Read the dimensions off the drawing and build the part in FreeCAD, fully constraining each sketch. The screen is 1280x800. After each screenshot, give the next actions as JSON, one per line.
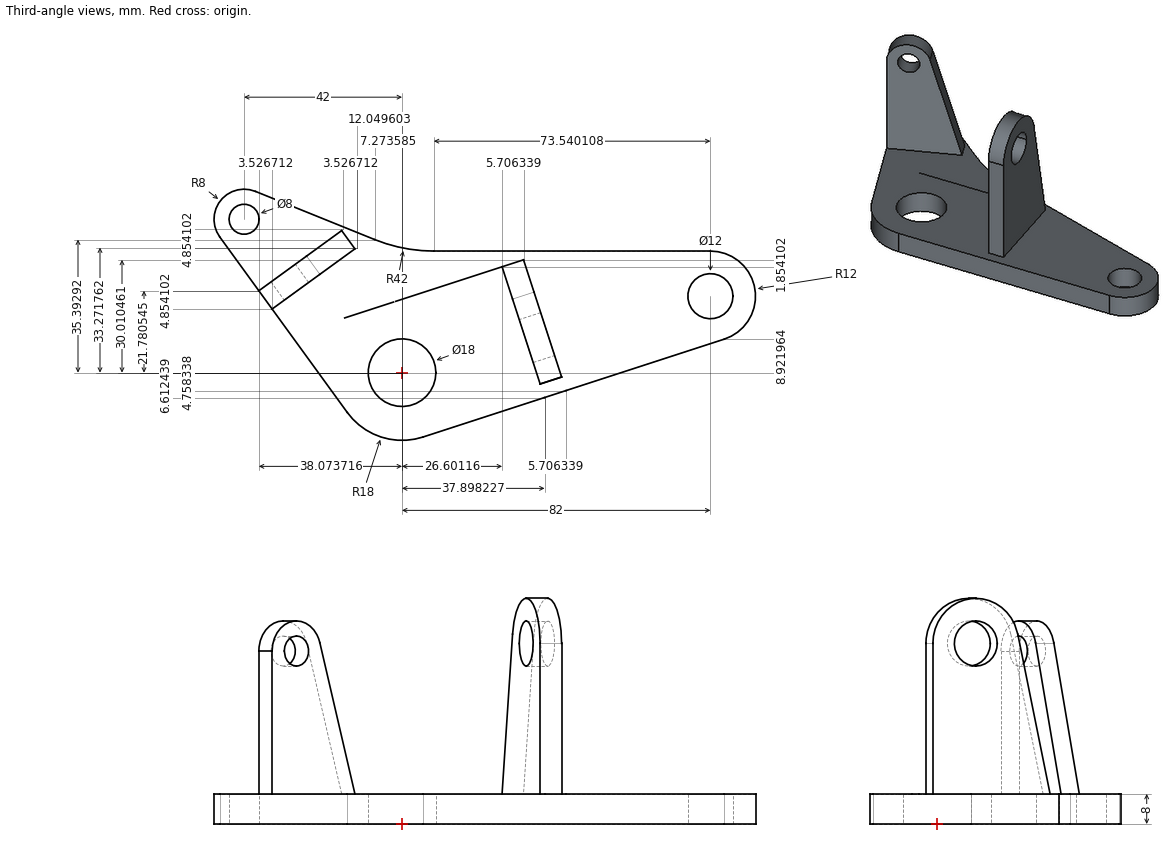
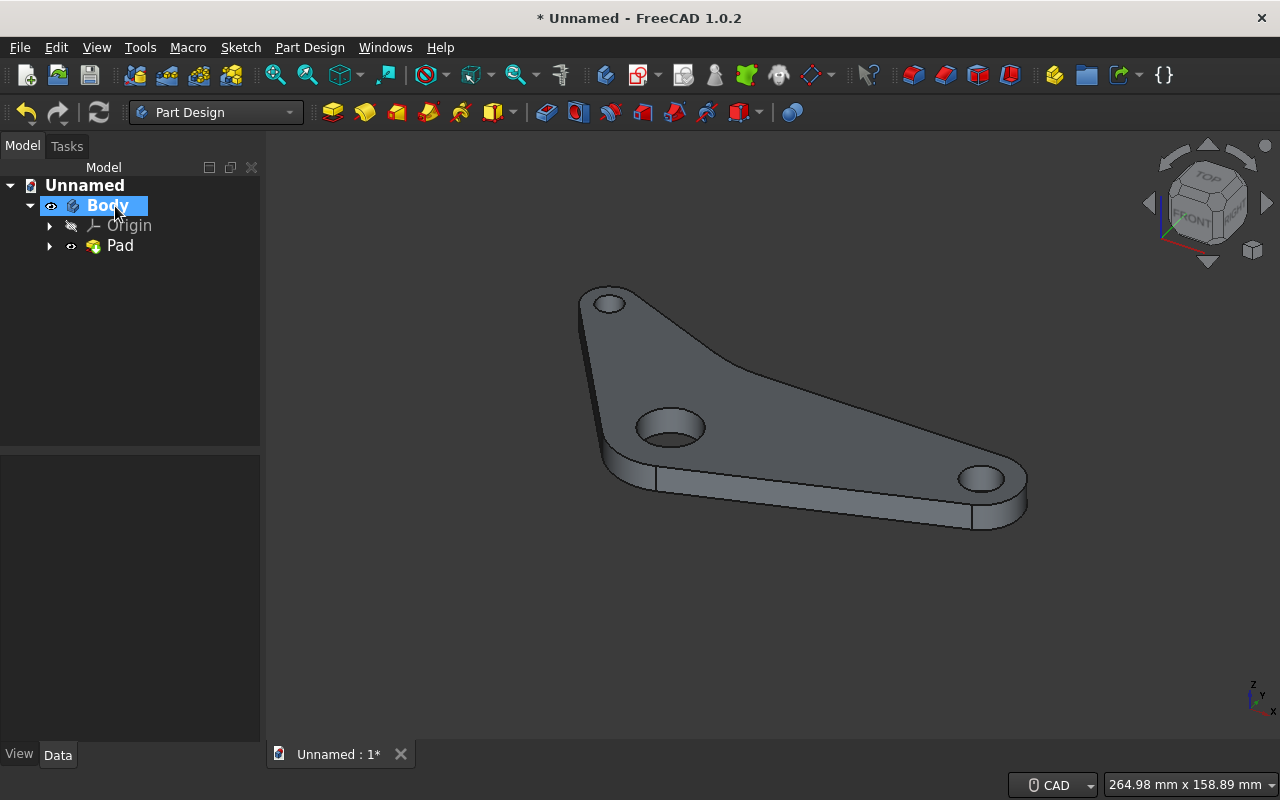
{"action": "left_click", "coordinate": [841, 444]}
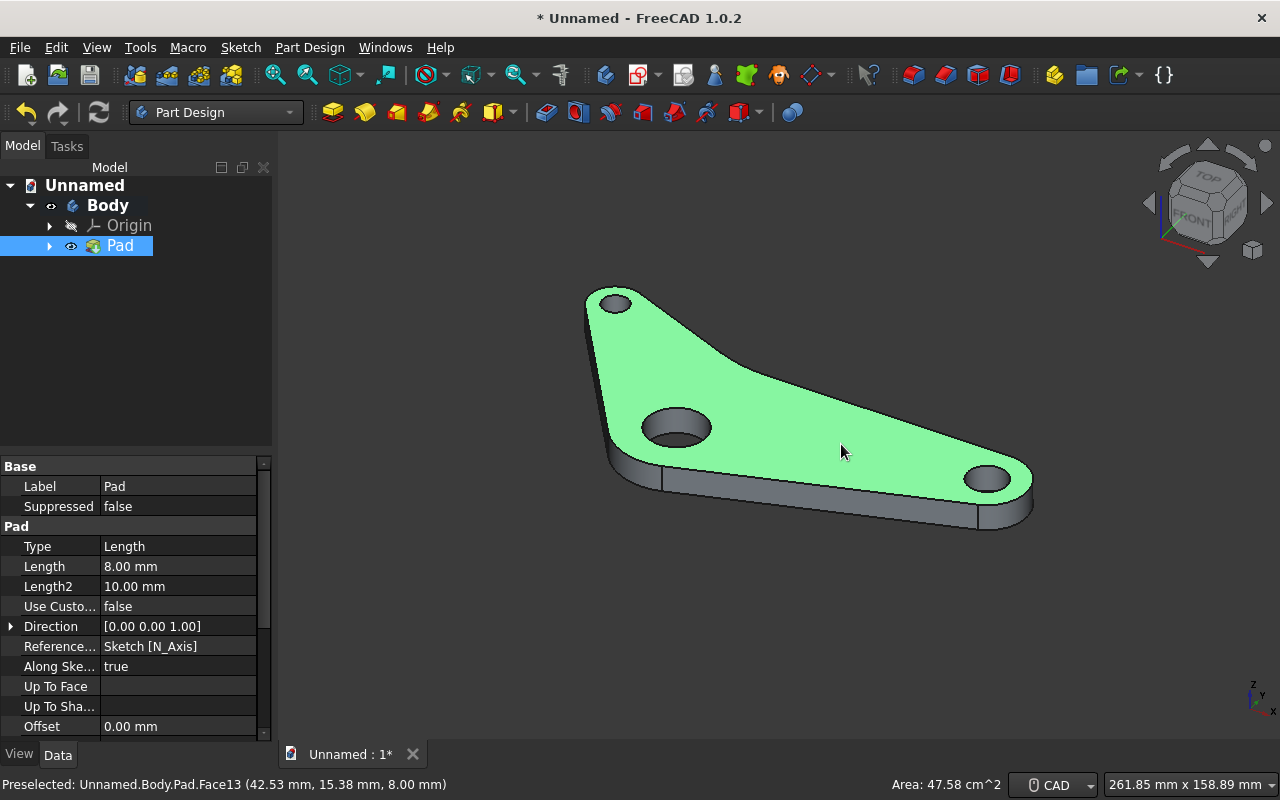
{"action": "left_click", "coordinate": [638, 76]}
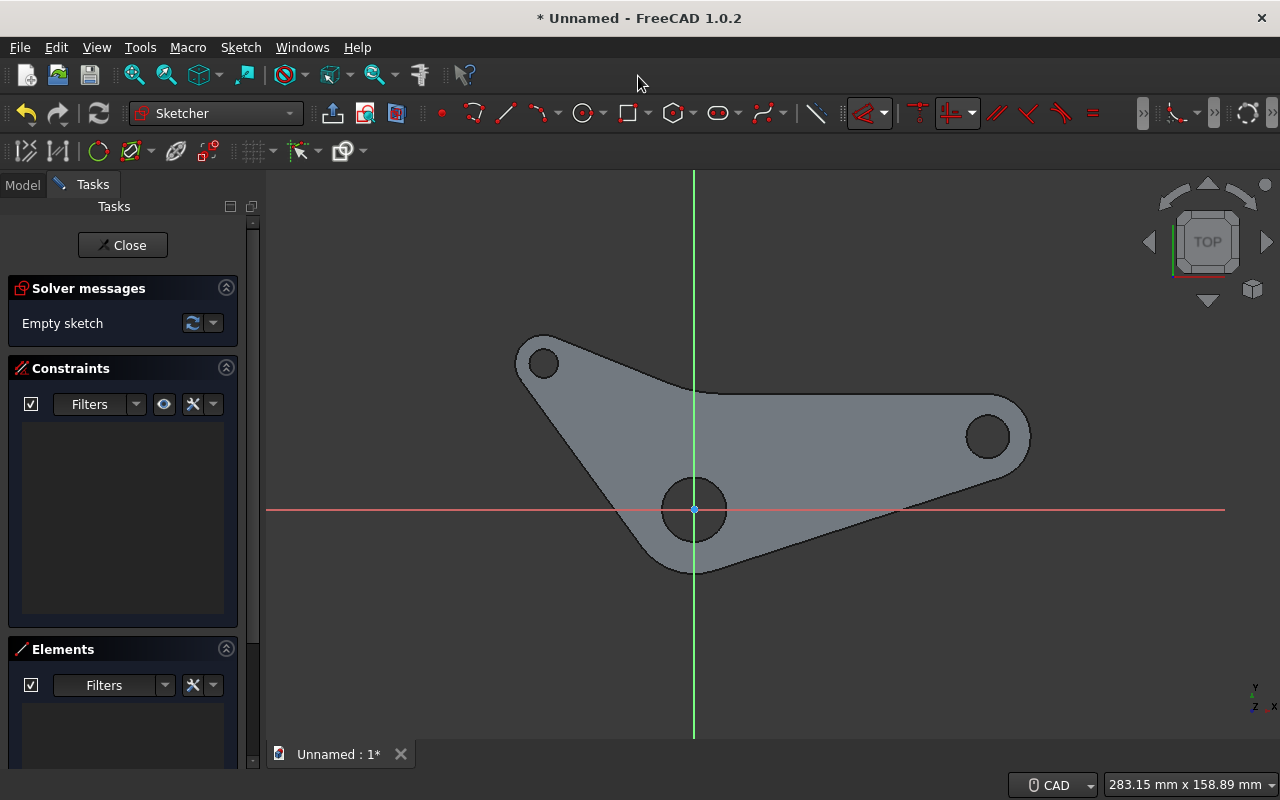
{"action": "scroll", "coordinate": [704, 452], "scroll_direction": "up", "scroll_amount": 3}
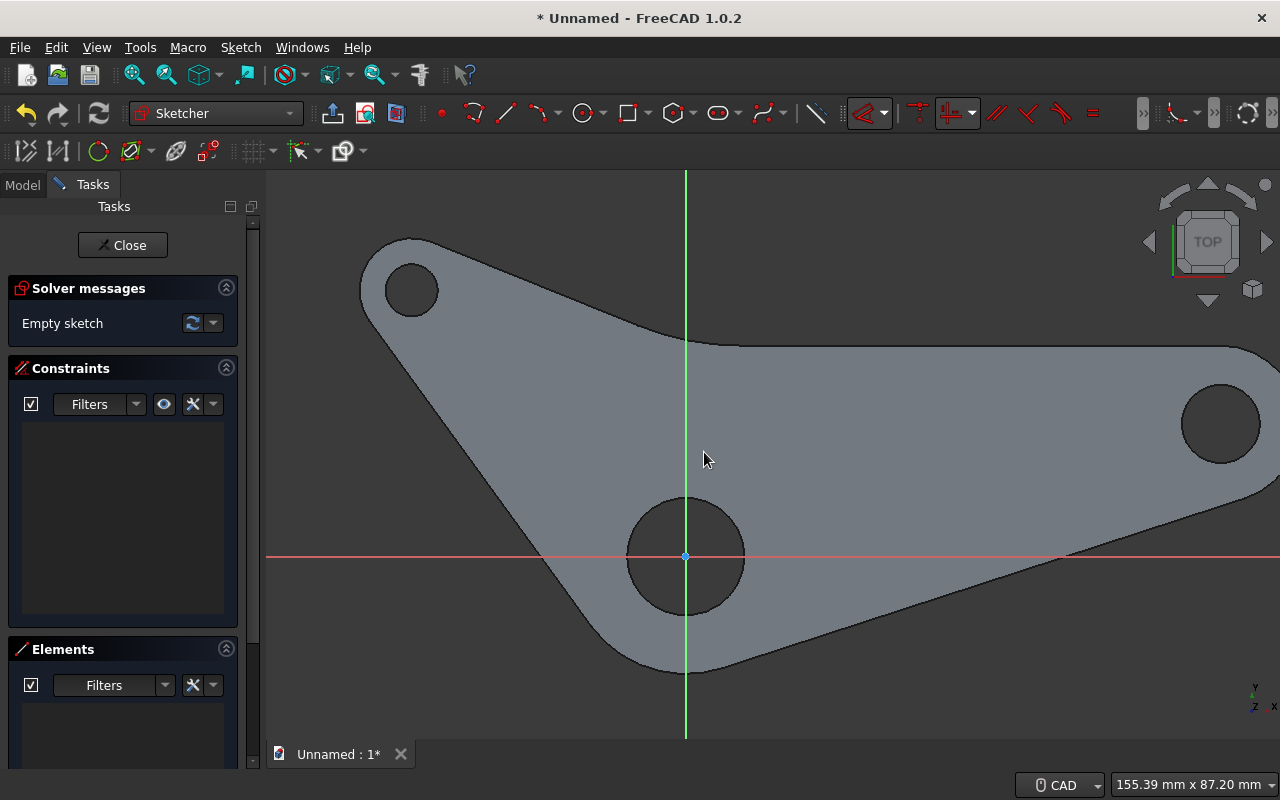
{"action": "key", "text": "g m"}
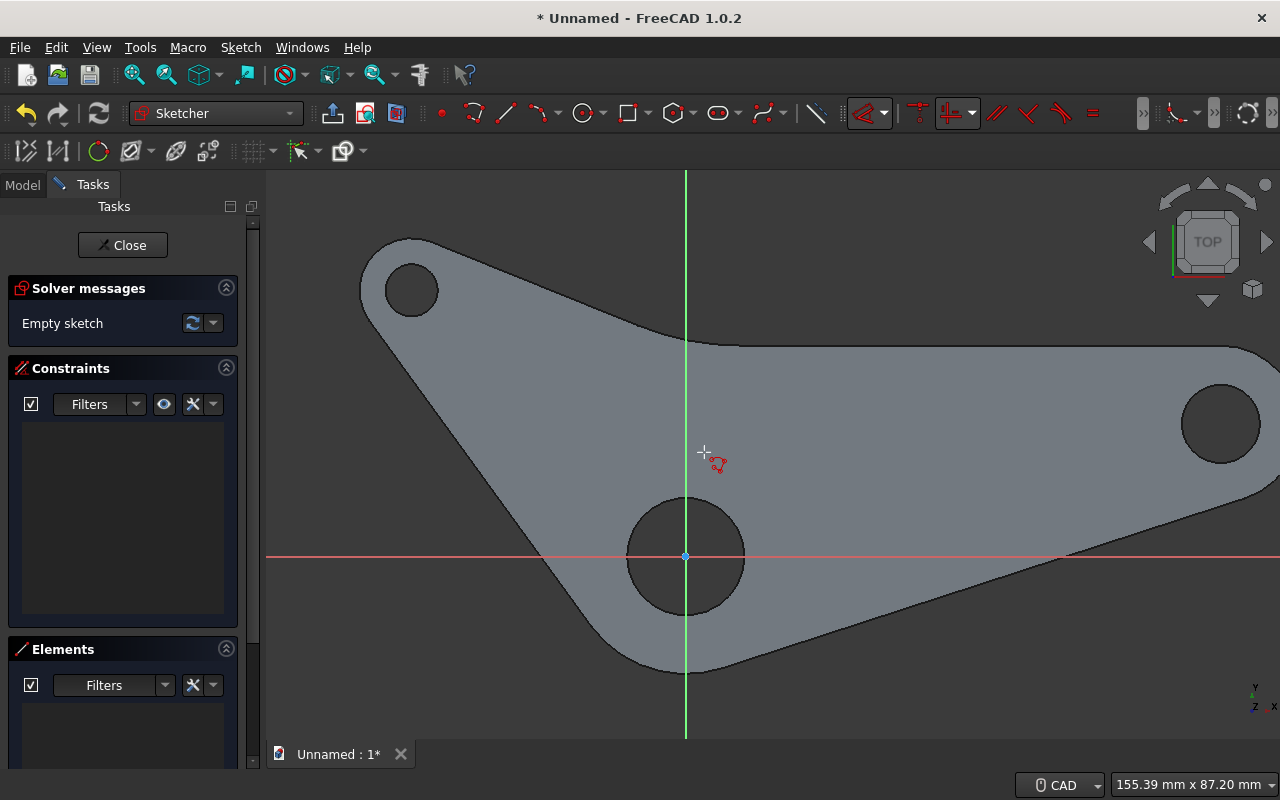
{"action": "left_click", "coordinate": [933, 600]}
{"action": "left_click", "coordinate": [970, 588]}
{"action": "left_click", "coordinate": [897, 361]}
{"action": "left_click", "coordinate": [859, 373]}
{"action": "left_click", "coordinate": [933, 601]}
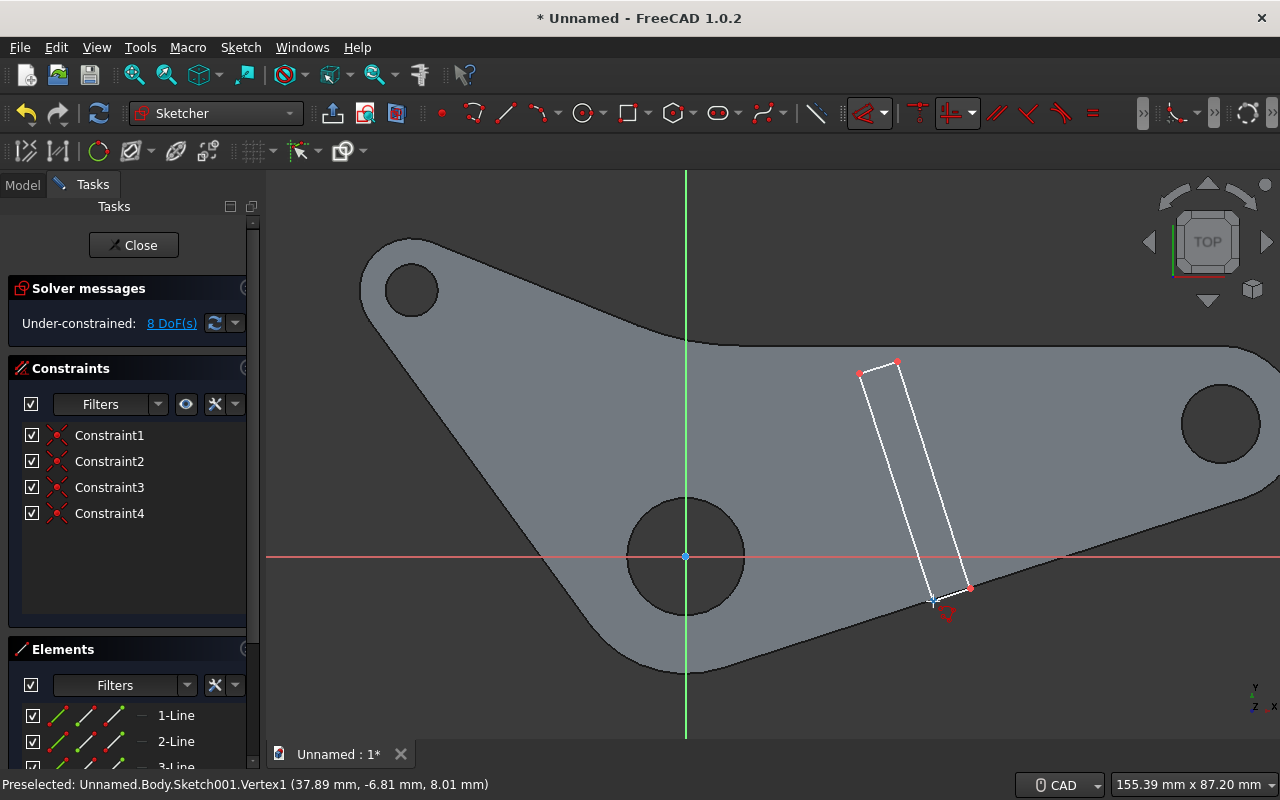
{"action": "left_click", "coordinate": [607, 339]}
{"action": "left_click", "coordinate": [584, 308]}
{"action": "left_click", "coordinate": [437, 414]}
{"action": "left_click", "coordinate": [460, 446]}
{"action": "left_click", "coordinate": [607, 340]}
{"action": "key", "text": "Escape"}
{"action": "key", "text": "Escape"}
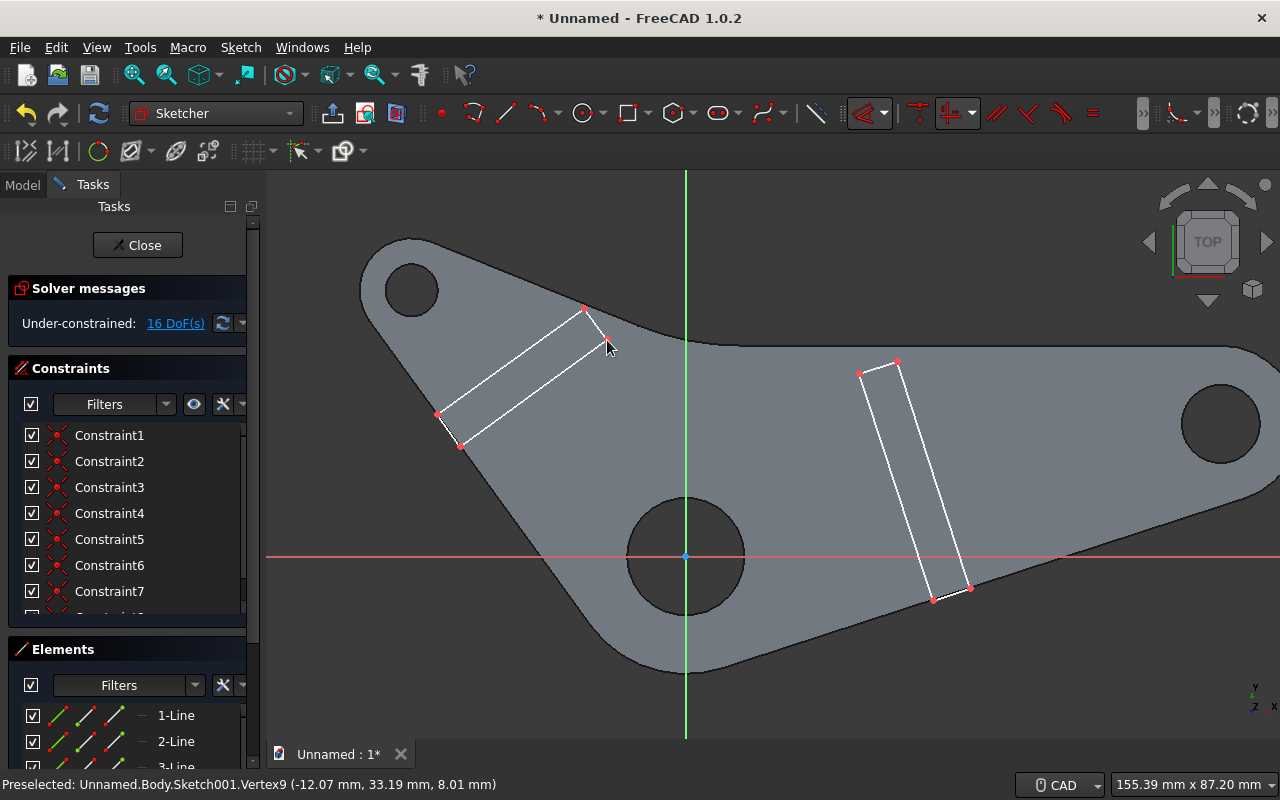
{"action": "left_click", "coordinate": [933, 601]}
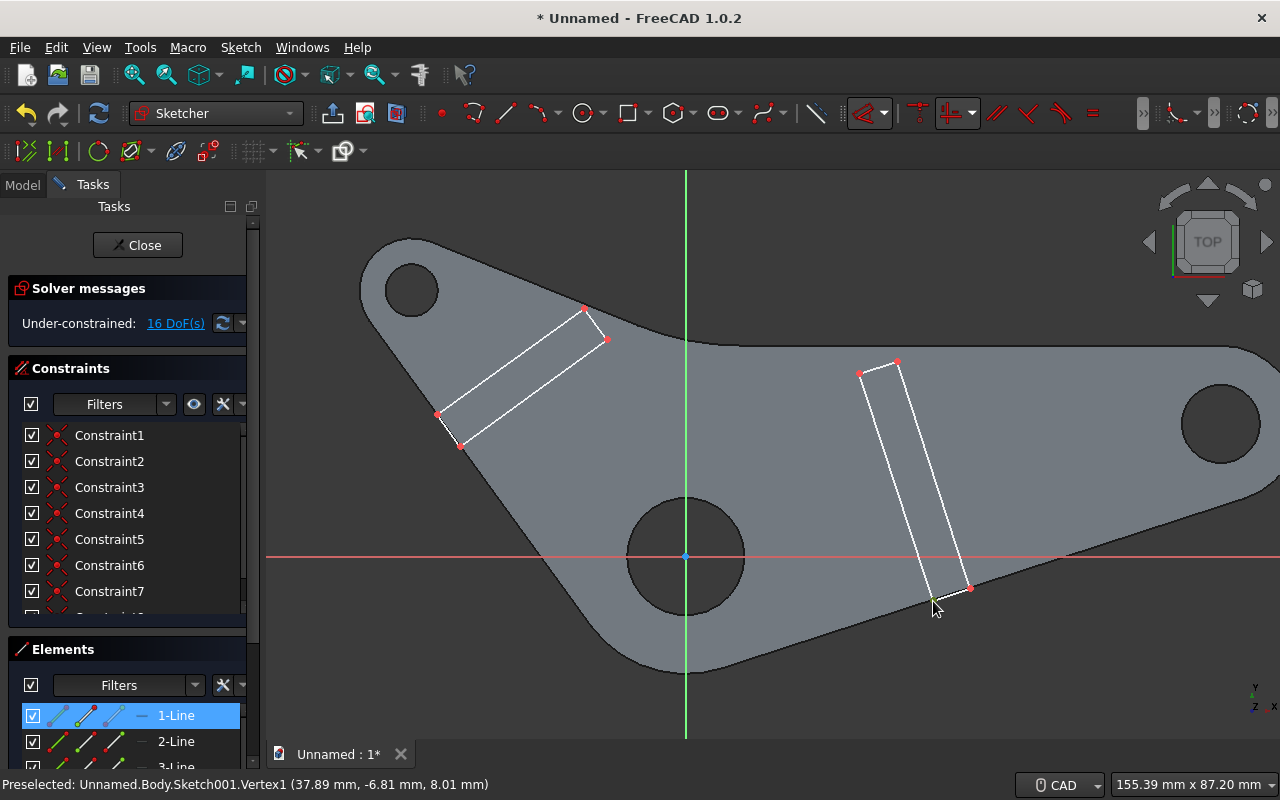
{"action": "key", "text": "i"}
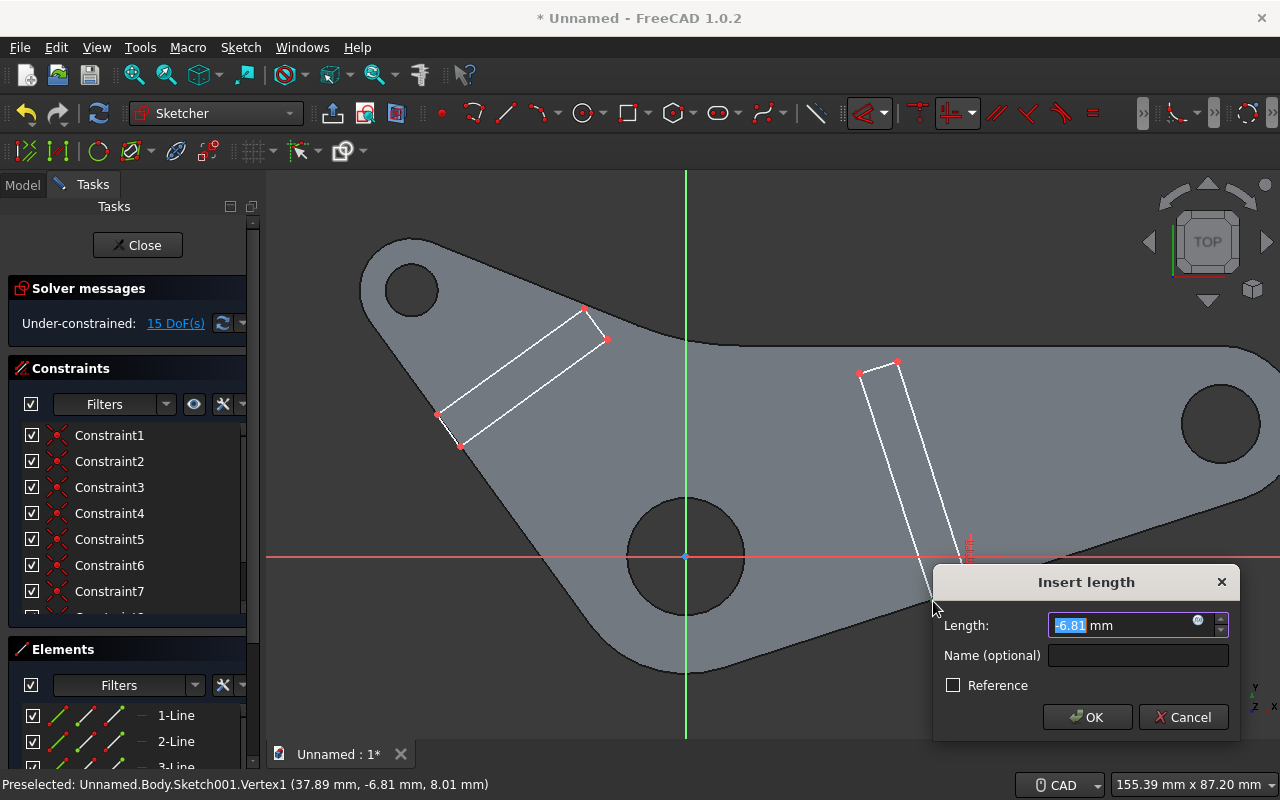
{"action": "type", "text": "-6.612439"}
{"action": "key", "text": "Return"}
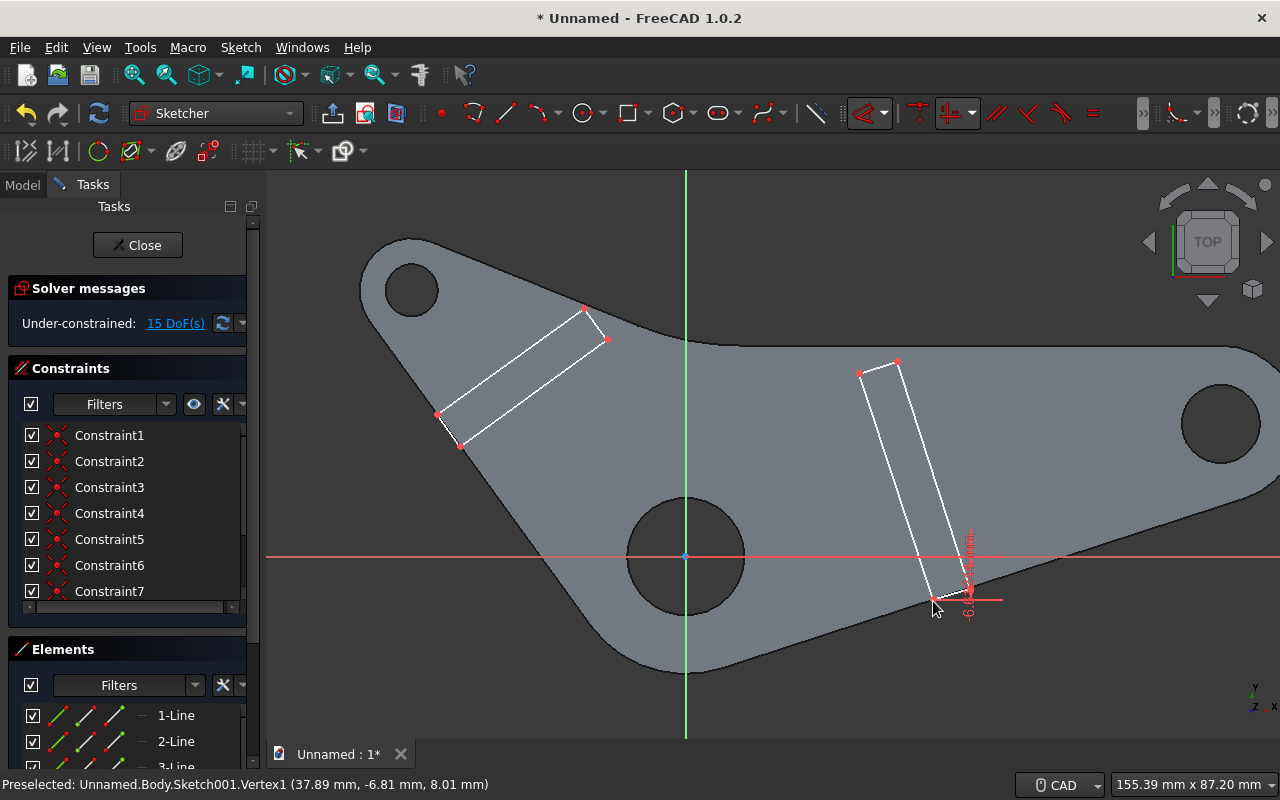
{"action": "scroll", "coordinate": [970, 589], "scroll_direction": "up", "scroll_amount": 2}